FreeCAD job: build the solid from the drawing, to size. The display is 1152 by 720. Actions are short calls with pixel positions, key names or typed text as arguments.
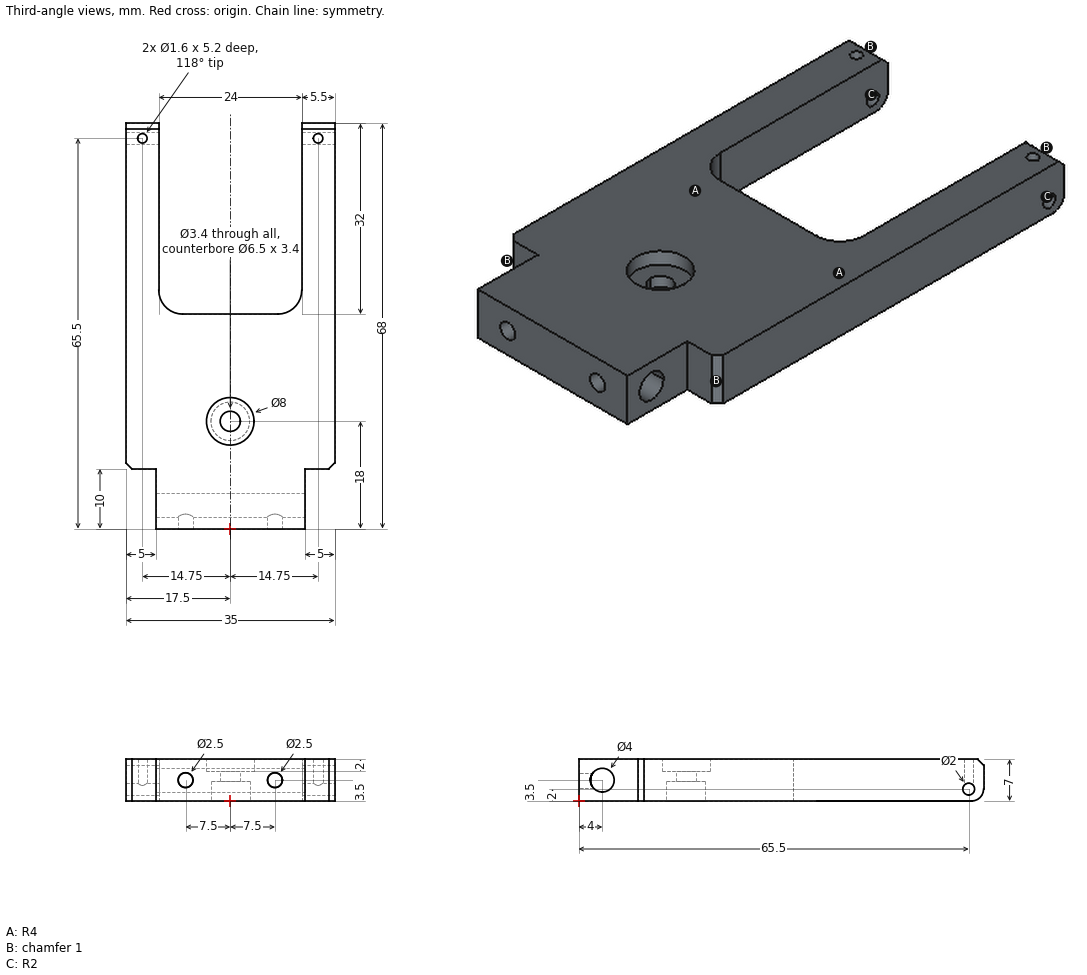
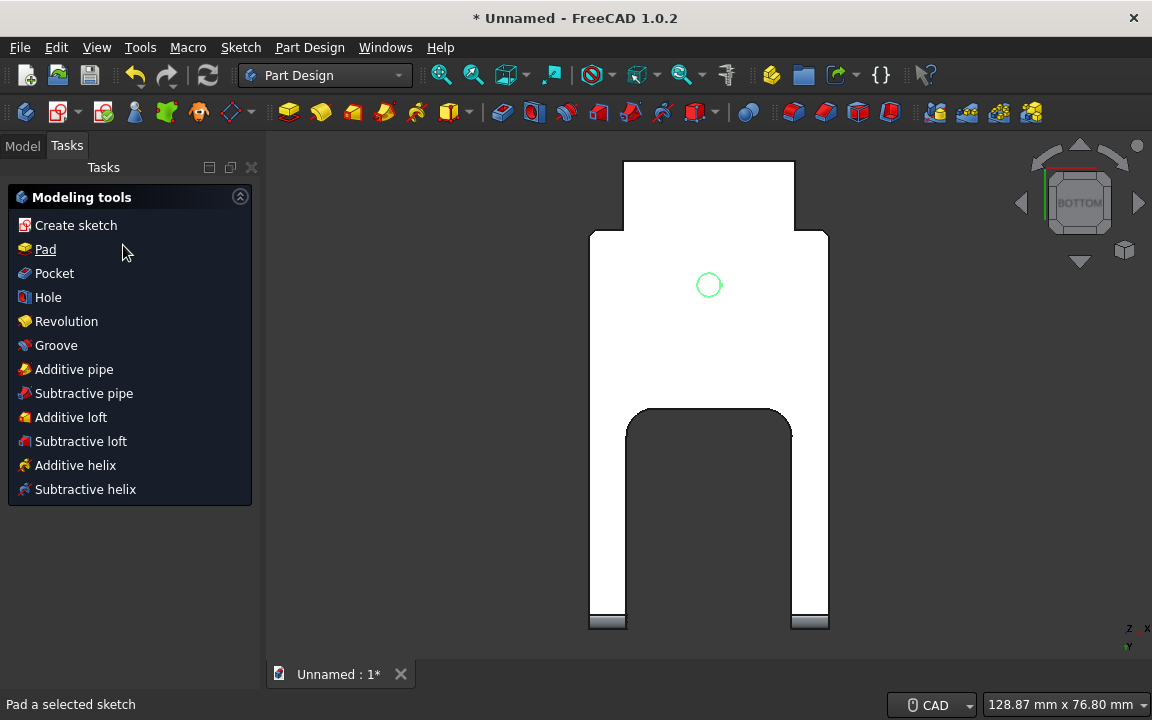
click(536, 112)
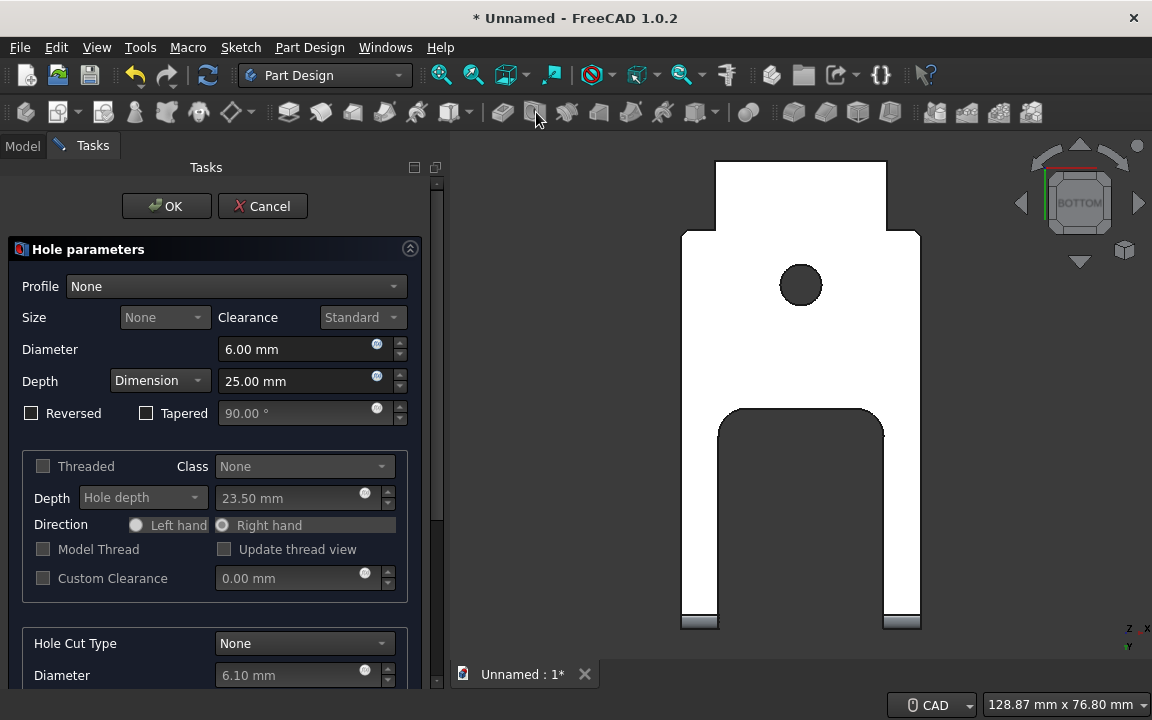
triple_click(305, 349)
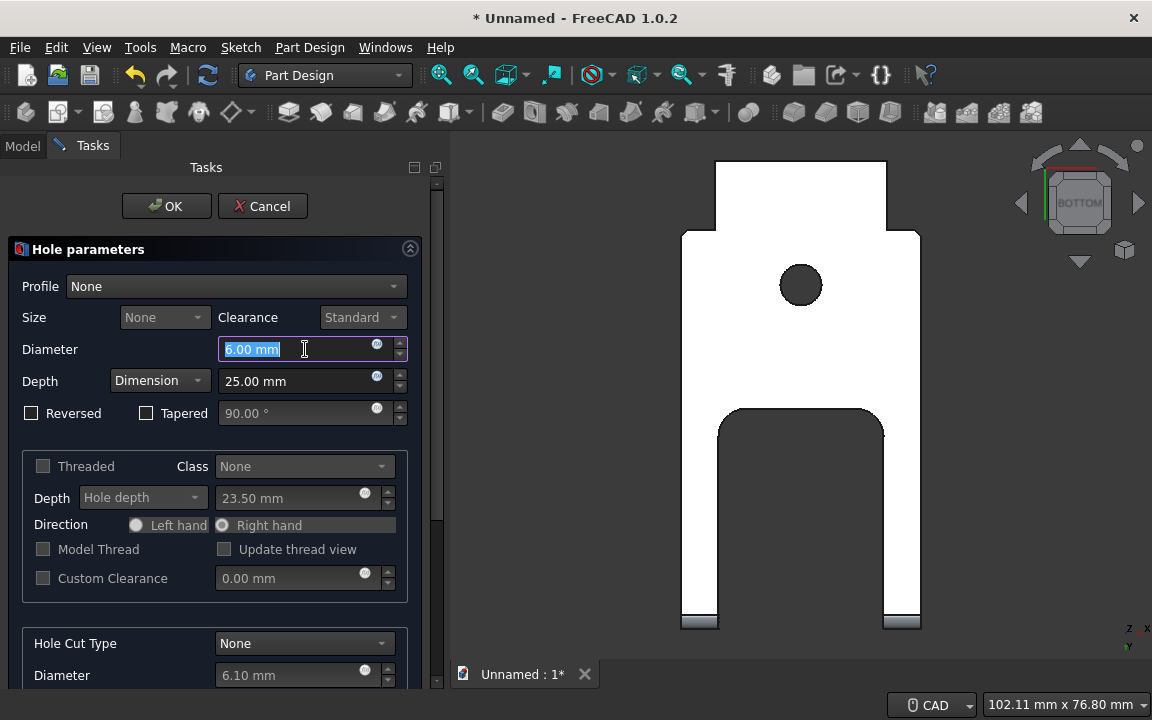
text(3.4)
key(Tab)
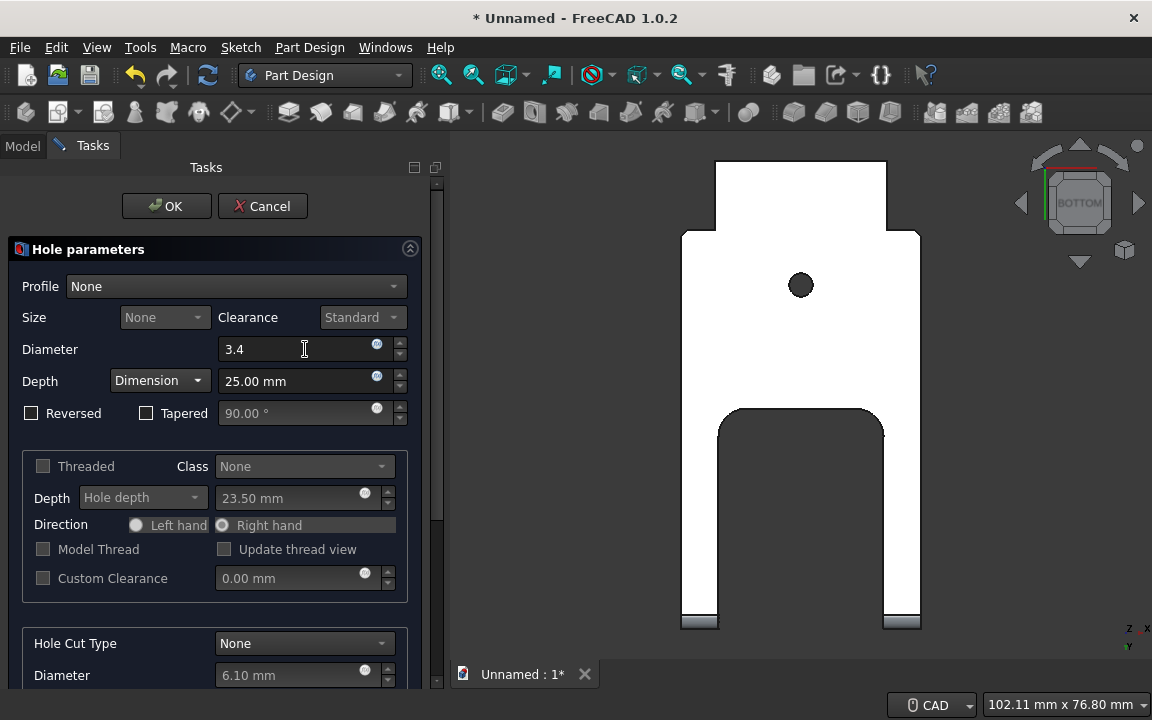
click(161, 380)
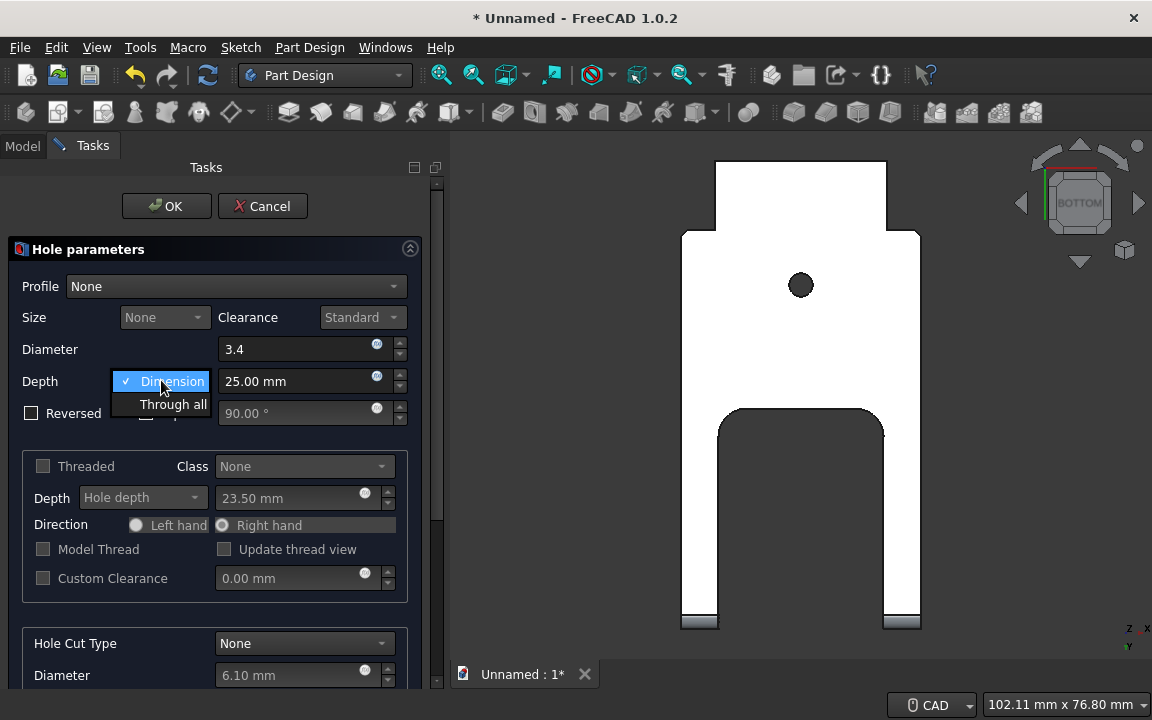
click(160, 404)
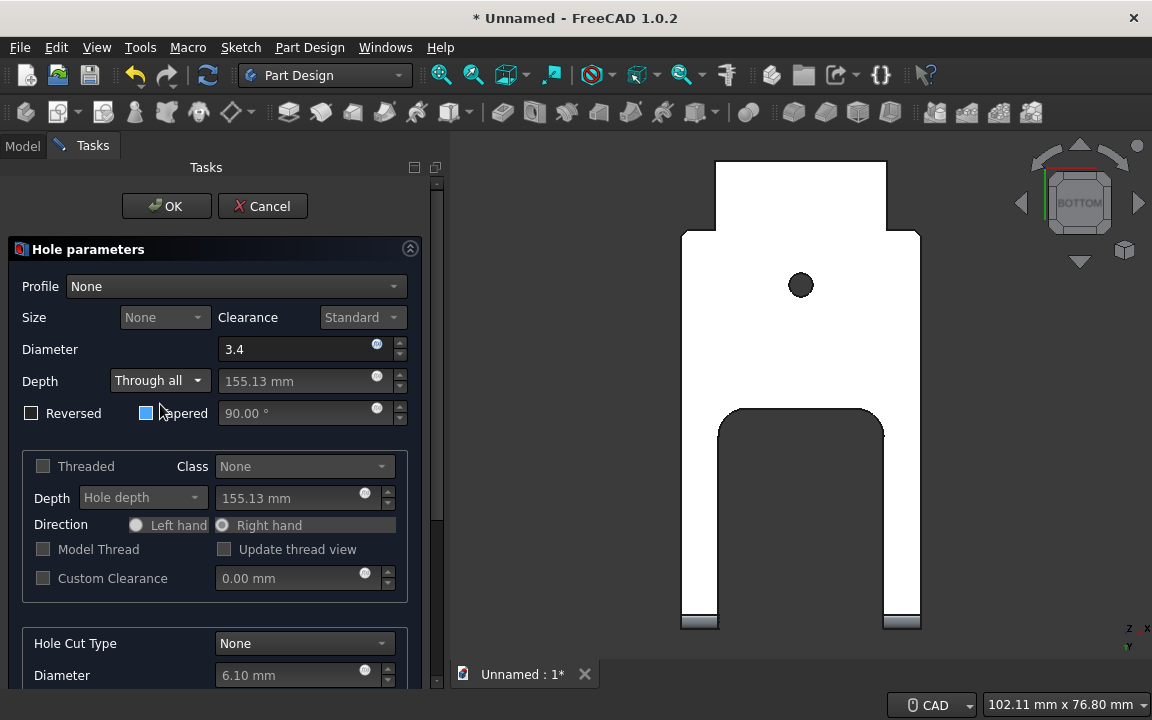
click(306, 644)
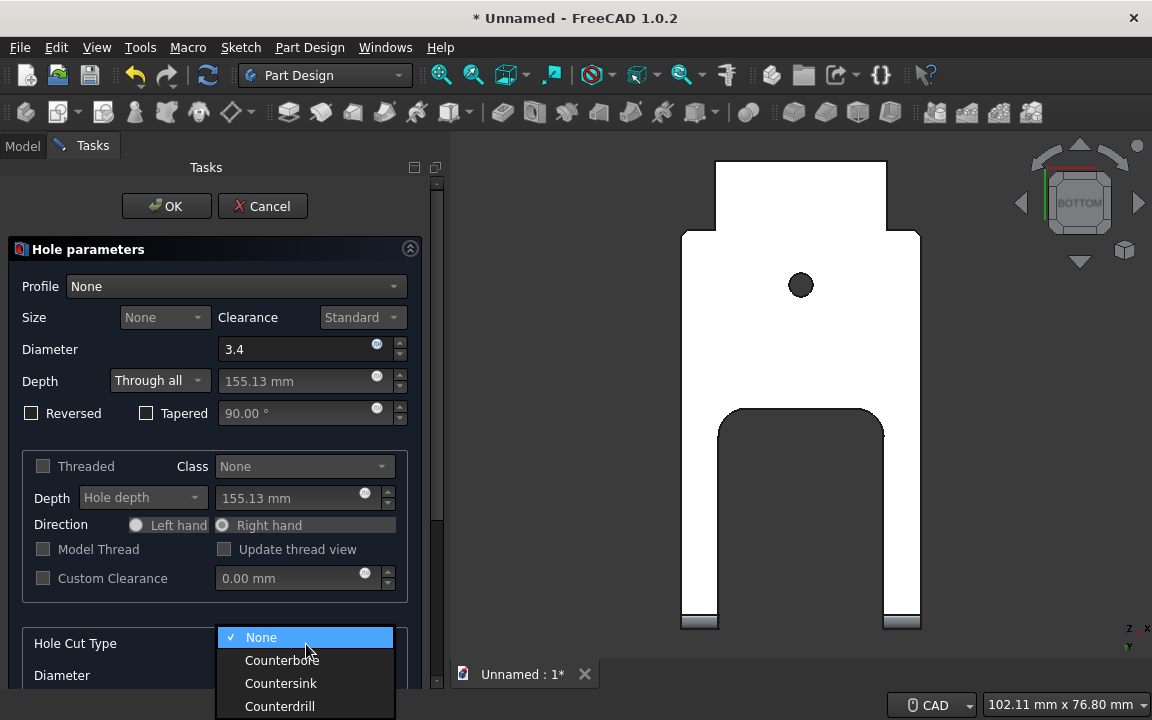
click(304, 660)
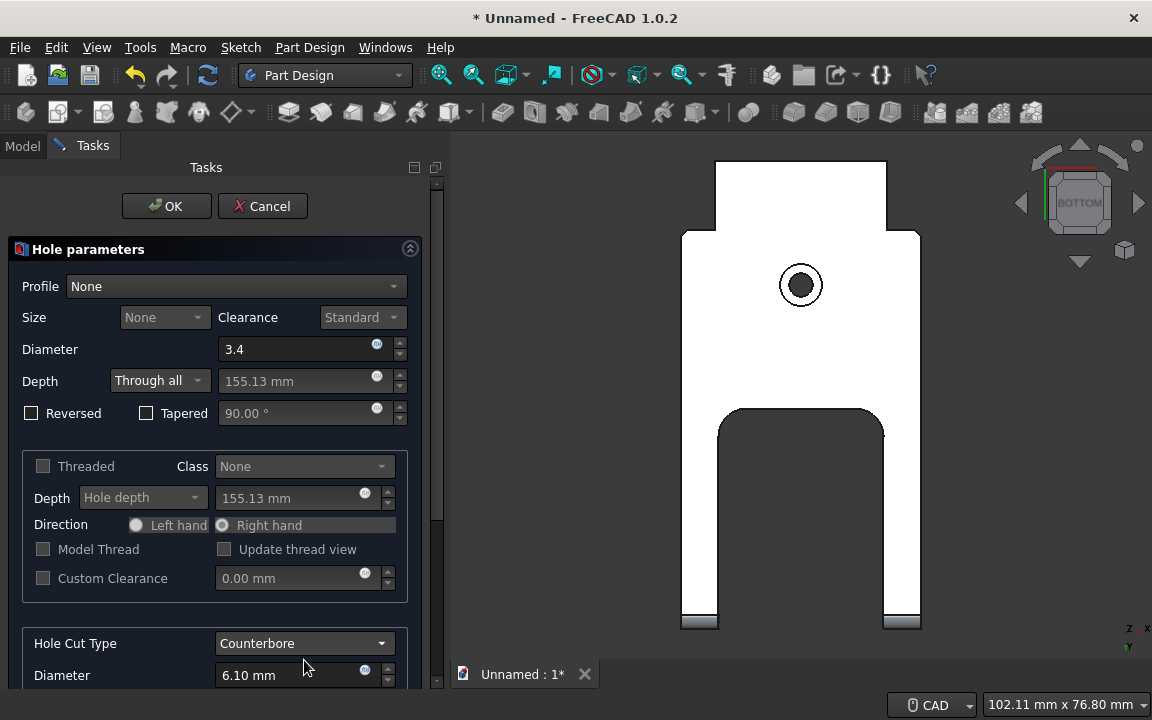
triple_click(298, 675)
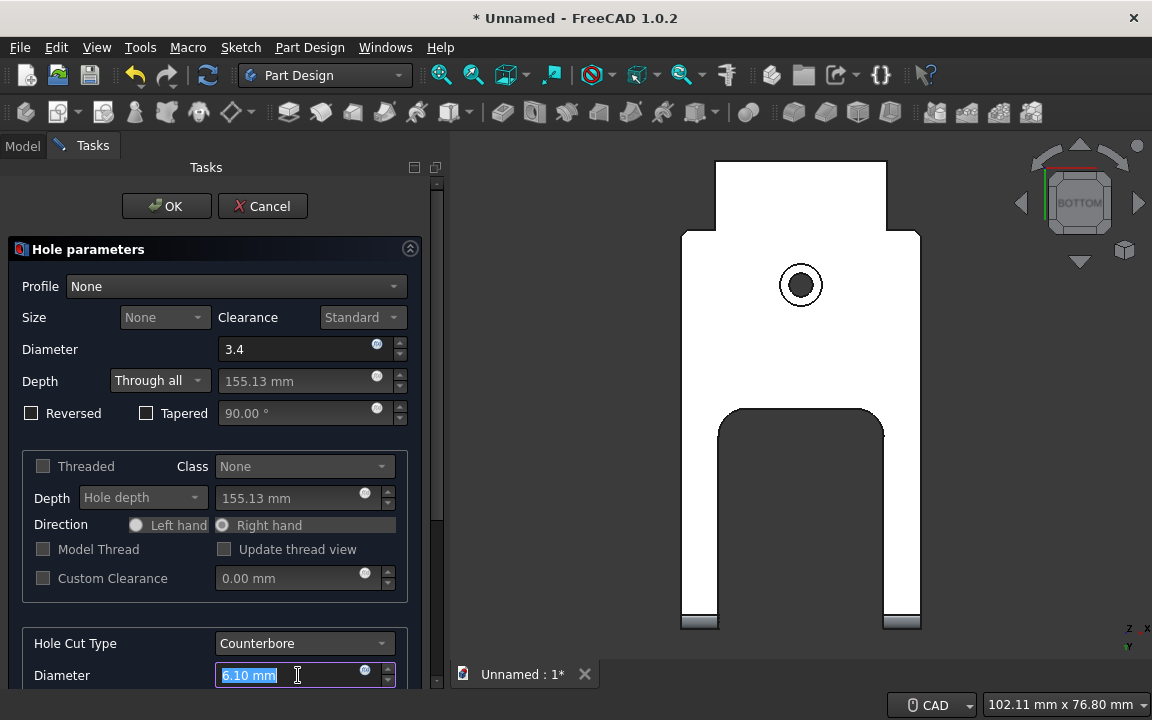
text(6.5)
key(Tab)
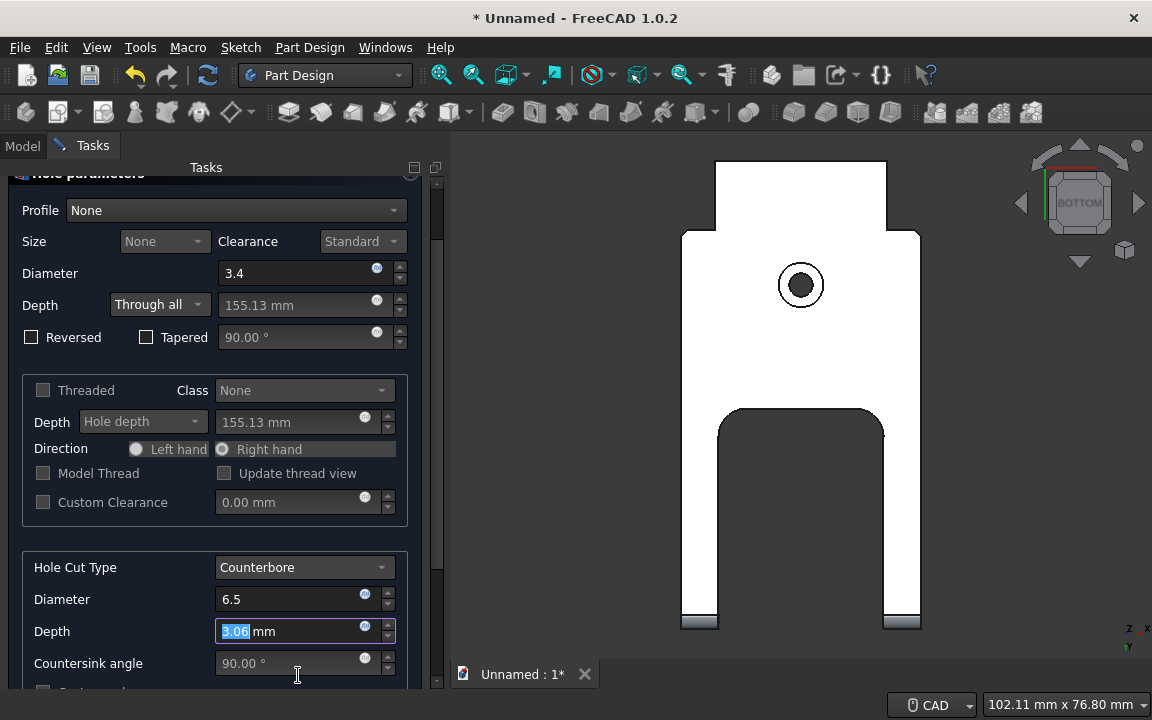
text(3.4)
key(Tab)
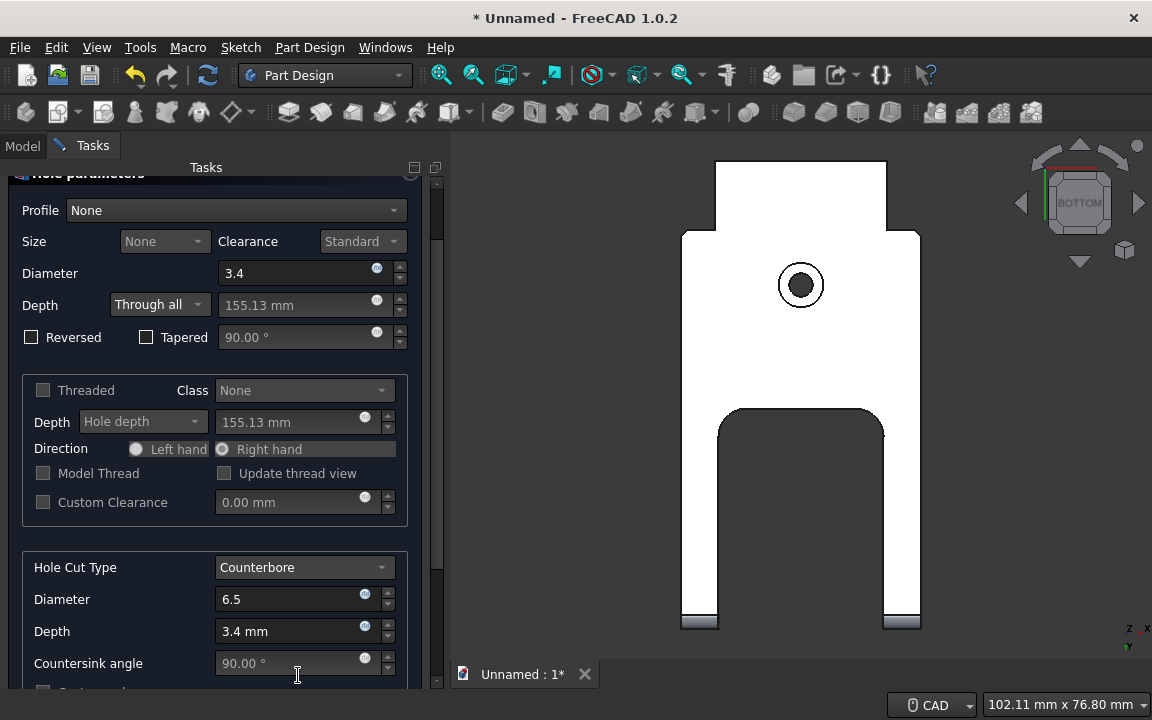
scroll(437, 432, up, 3)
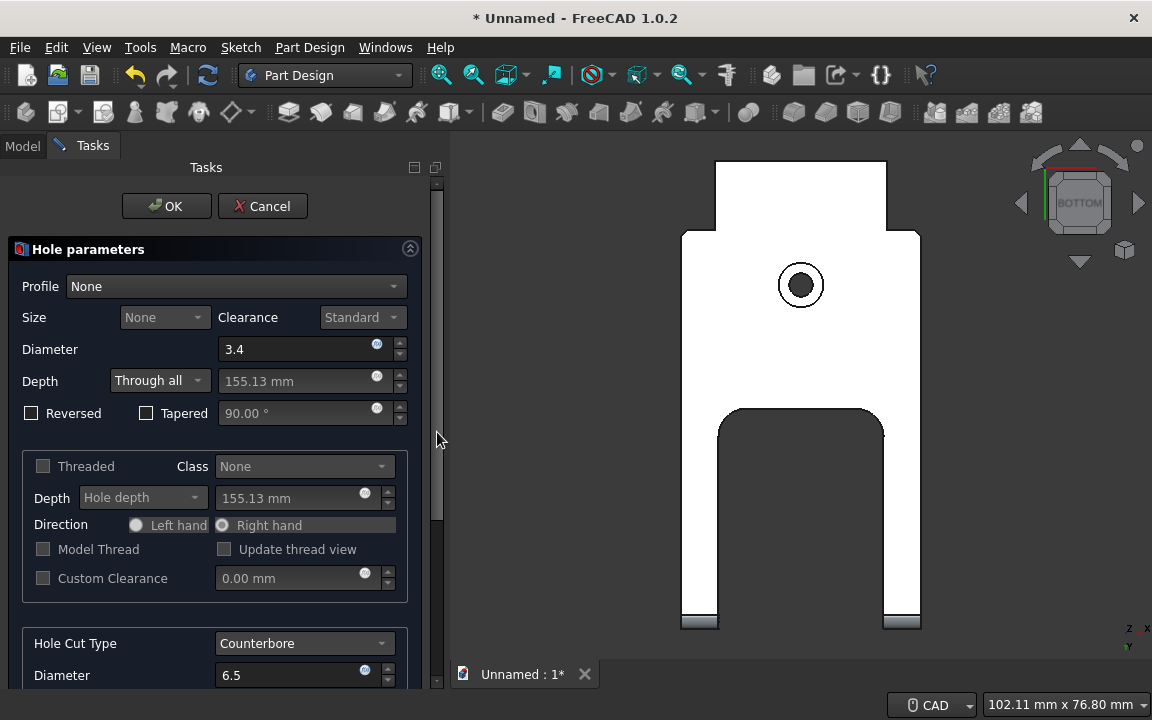
click(167, 206)